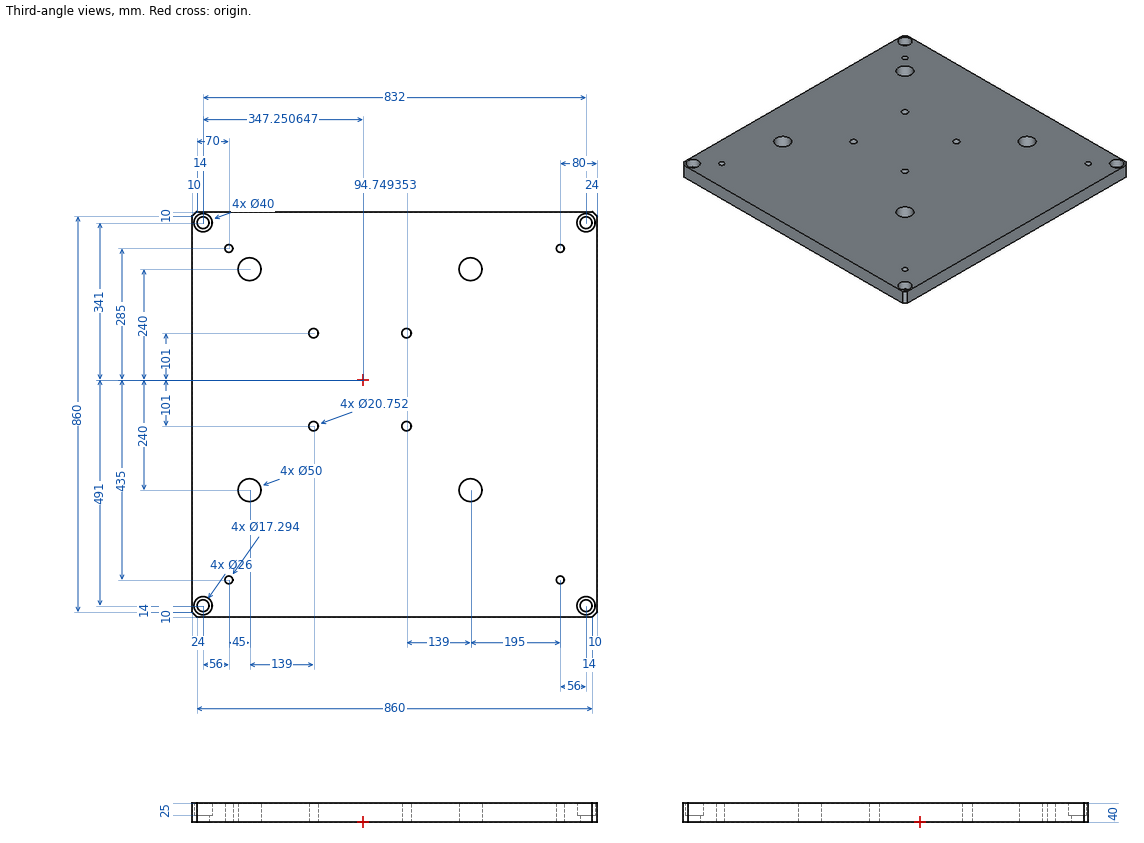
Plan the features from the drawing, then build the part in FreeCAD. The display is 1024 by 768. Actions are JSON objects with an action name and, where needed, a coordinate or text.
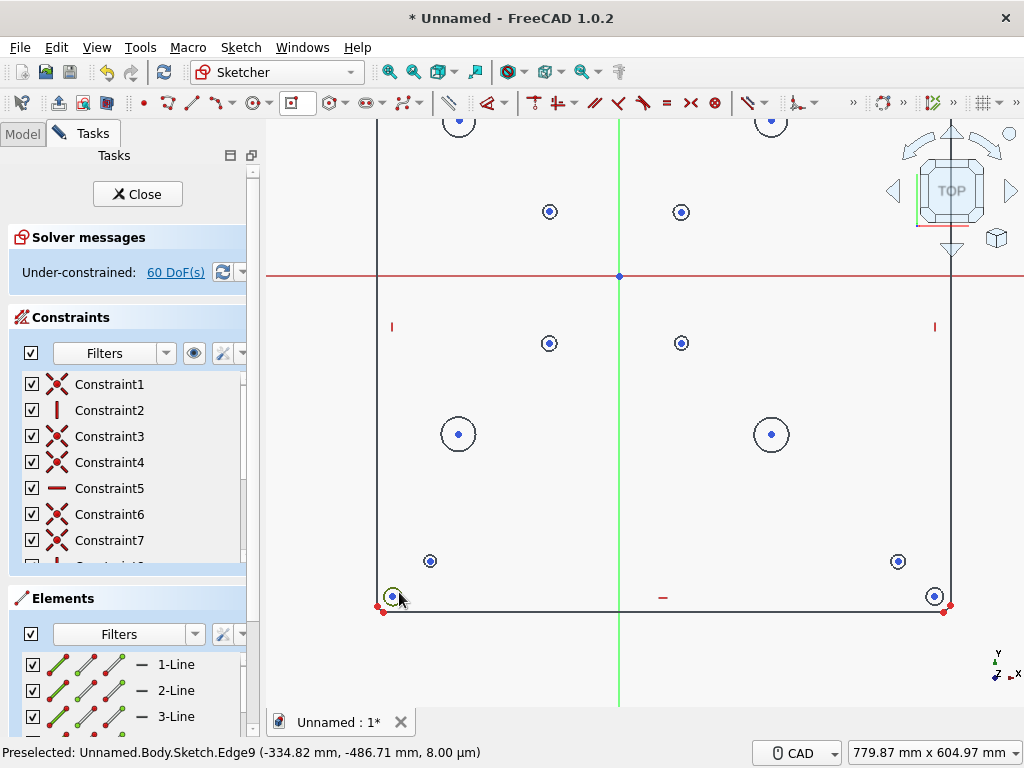
{"action": "scroll", "coordinate": [762, 591], "scroll_direction": "up", "scroll_amount": 5}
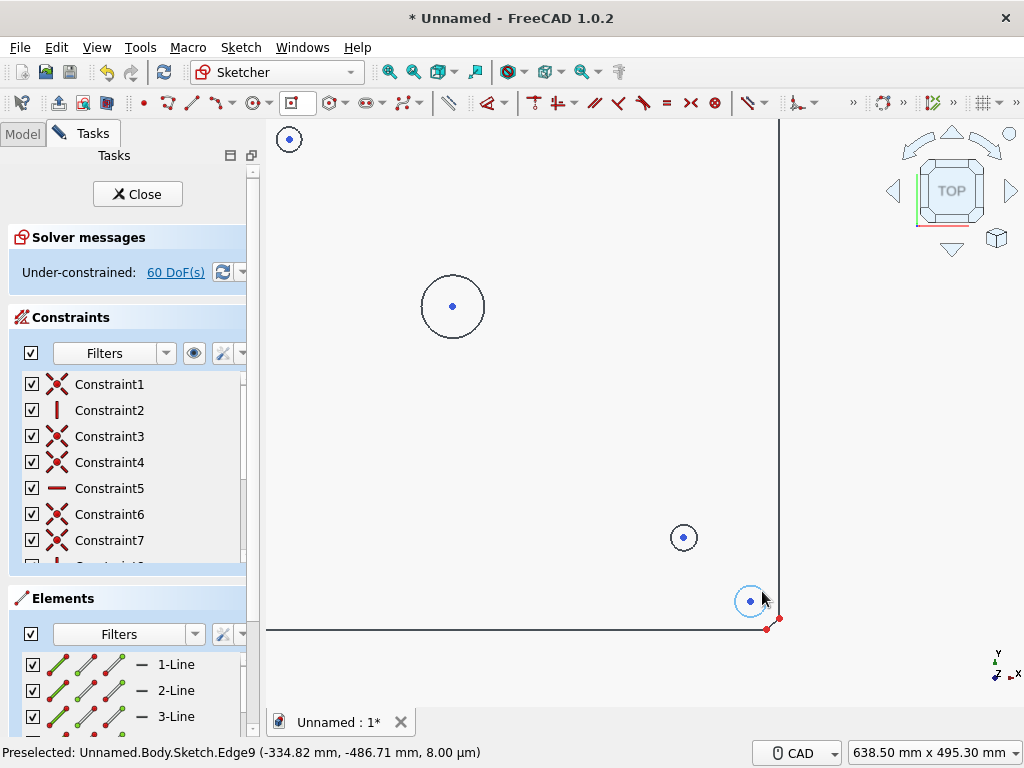
{"action": "left_click", "coordinate": [762, 590]}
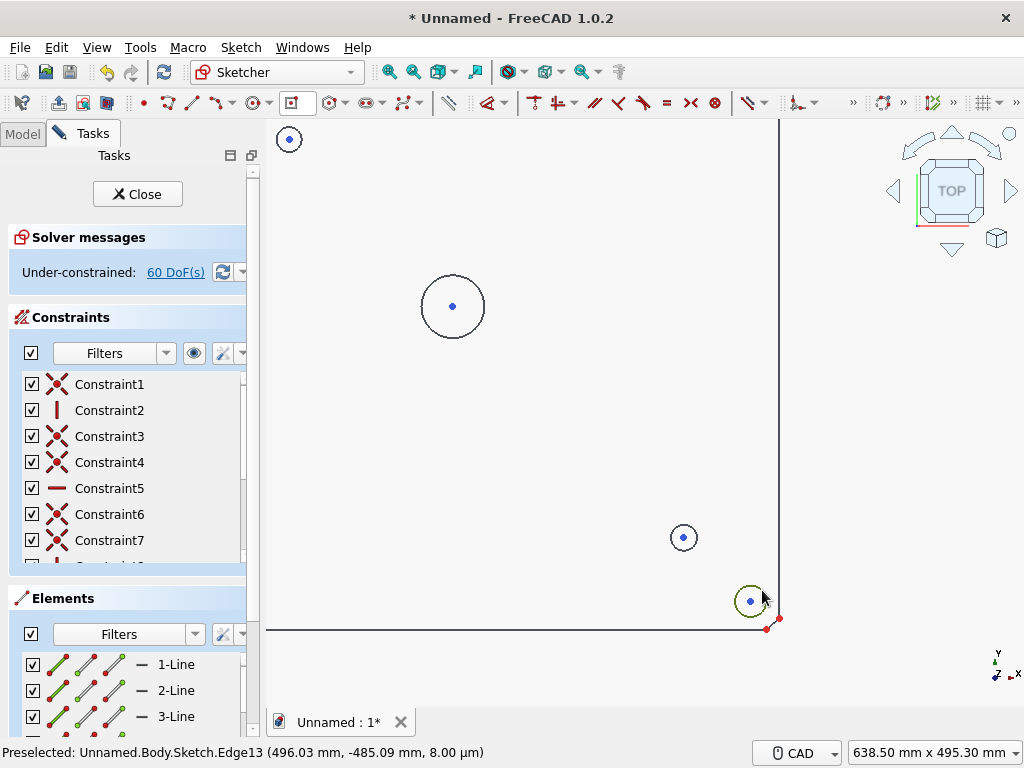
{"action": "scroll", "coordinate": [762, 591], "scroll_direction": "down", "scroll_amount": 5}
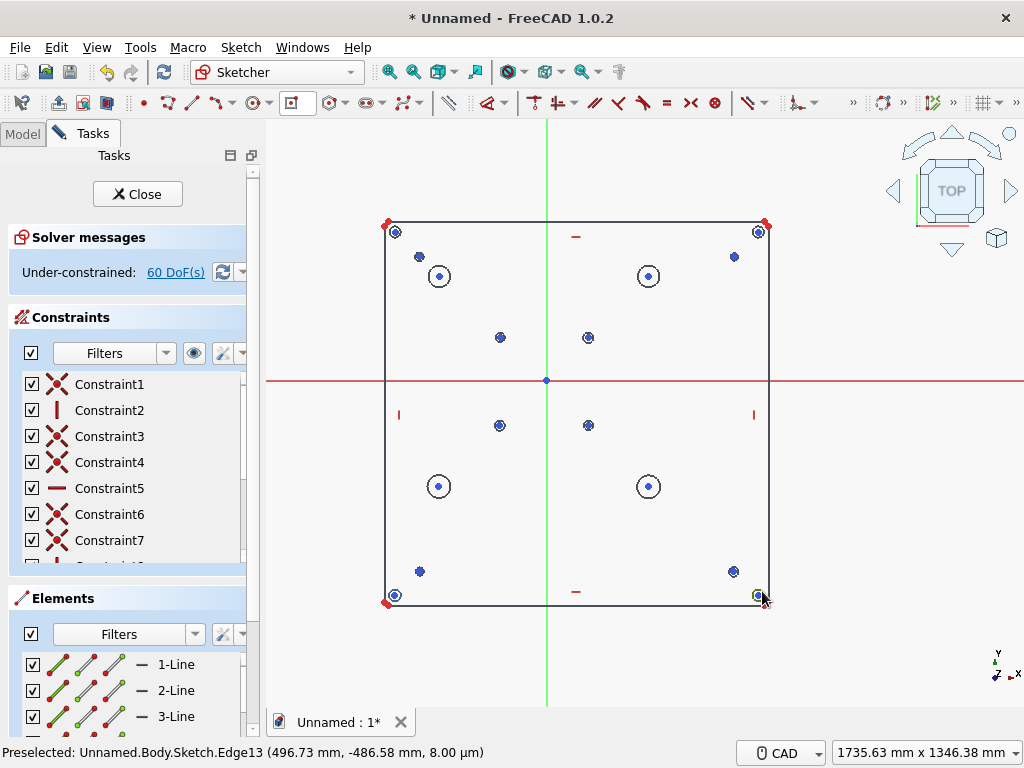
{"action": "scroll", "coordinate": [399, 228], "scroll_direction": "up", "scroll_amount": 5}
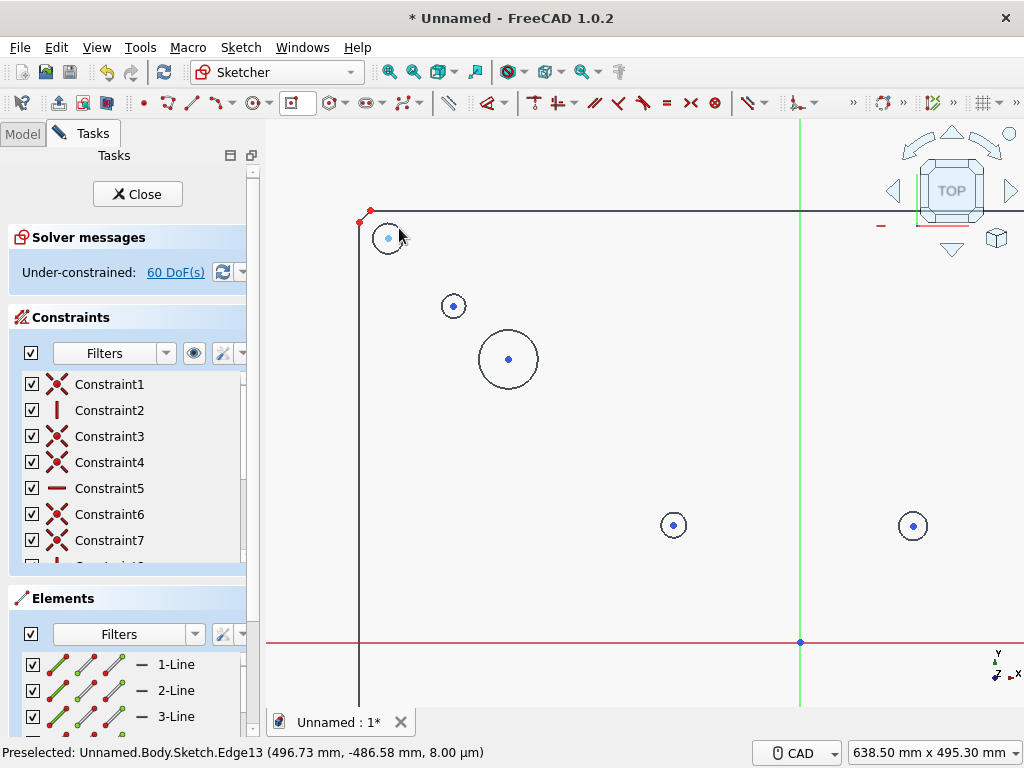
{"action": "left_click", "coordinate": [399, 228]}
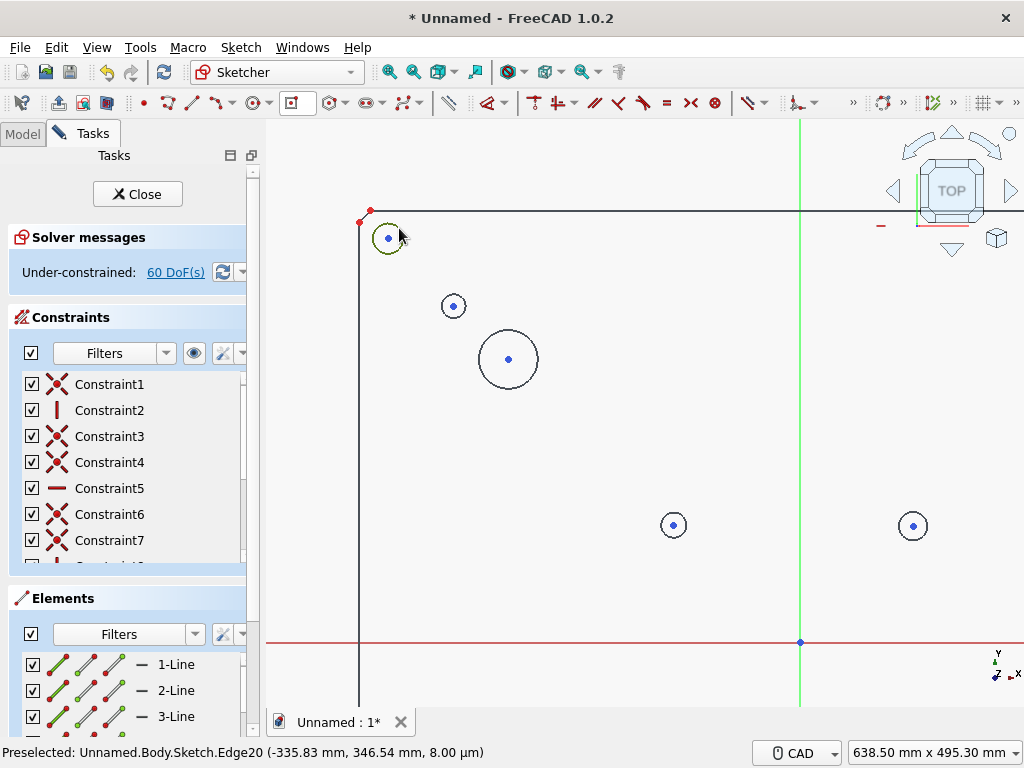
{"action": "scroll", "coordinate": [399, 227], "scroll_direction": "down", "scroll_amount": 5}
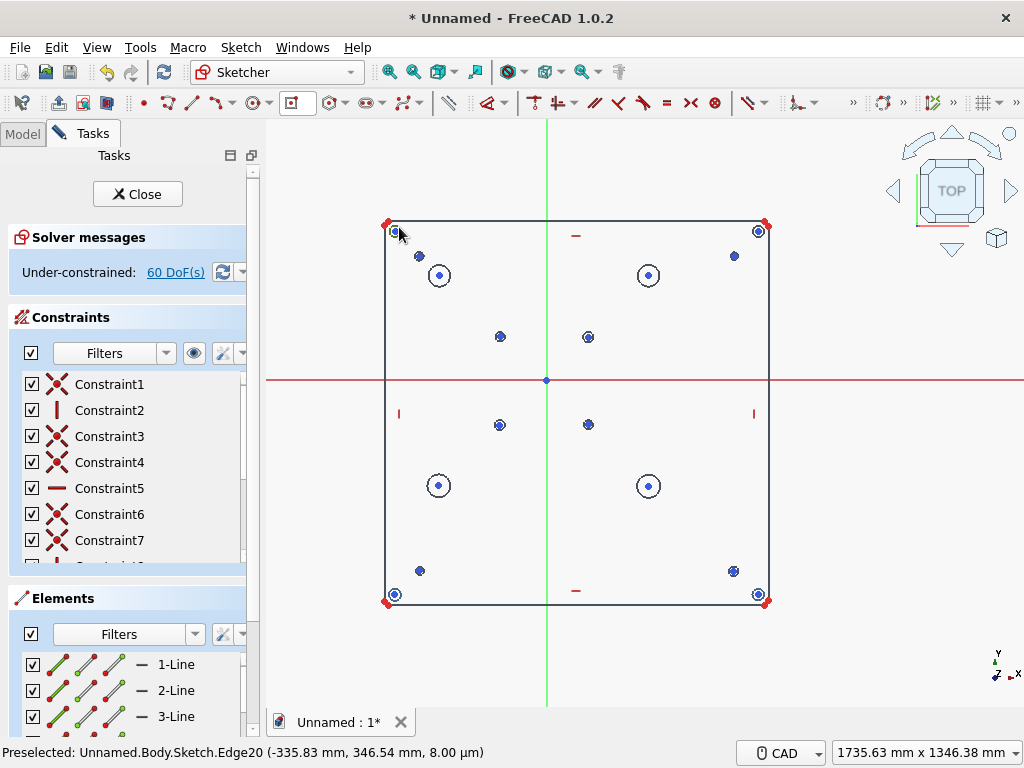
{"action": "scroll", "coordinate": [762, 227], "scroll_direction": "up", "scroll_amount": 5}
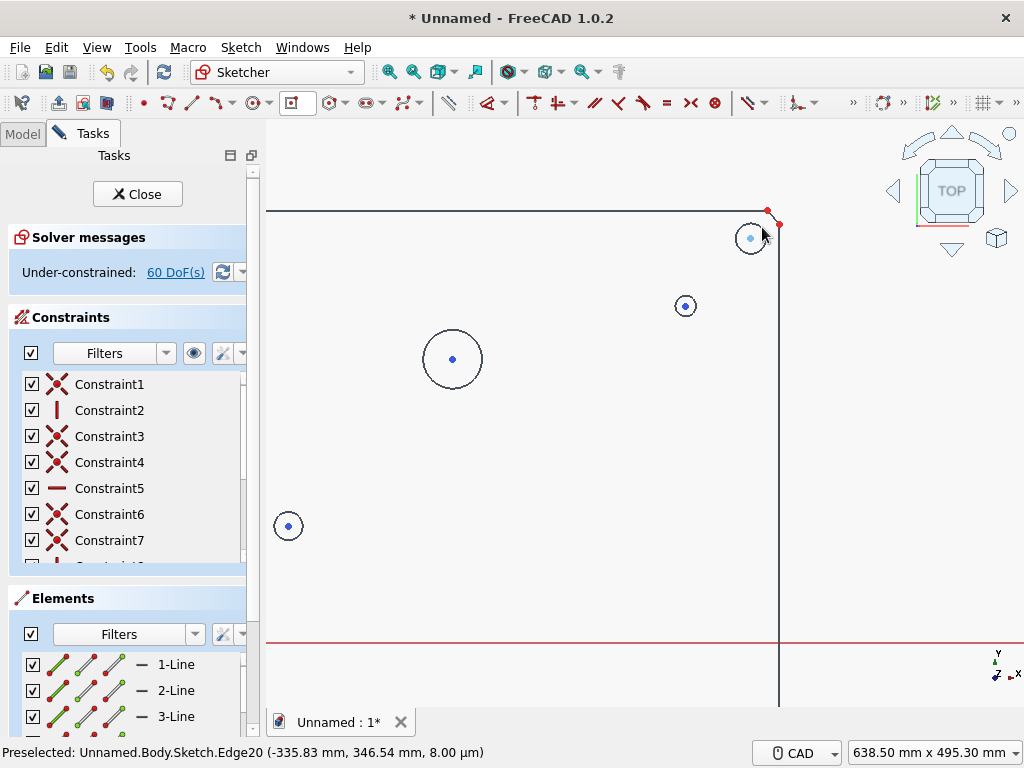
{"action": "left_click", "coordinate": [762, 228]}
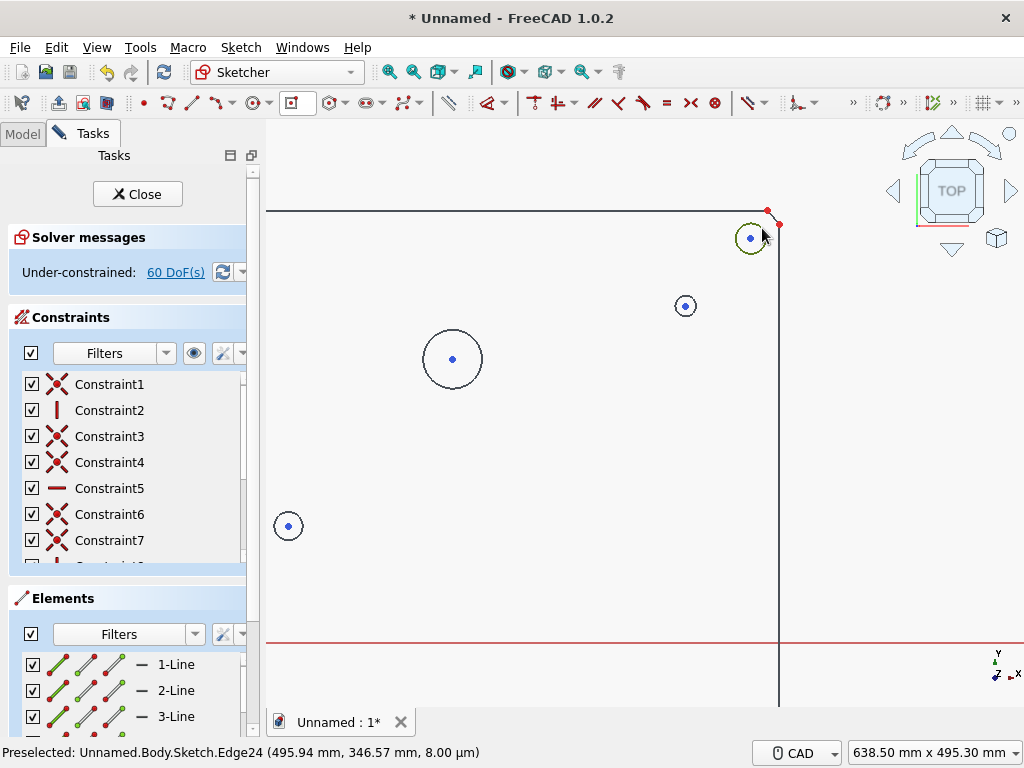
{"action": "key", "text": "e"}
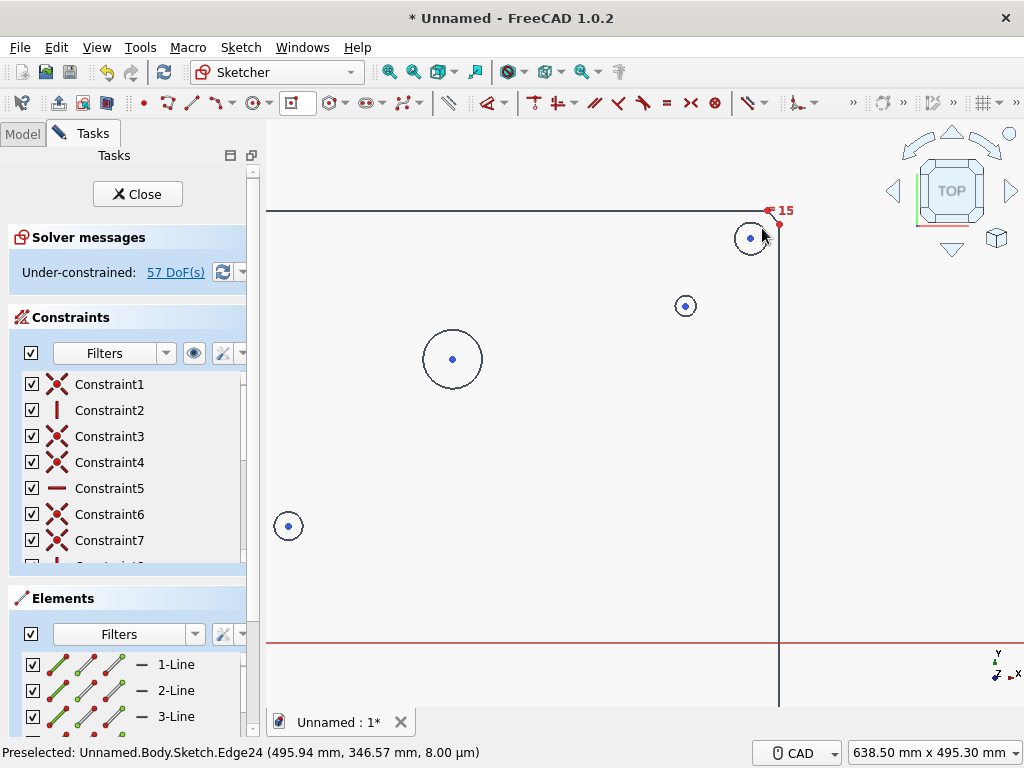
{"action": "scroll", "coordinate": [762, 227], "scroll_direction": "down", "scroll_amount": 5}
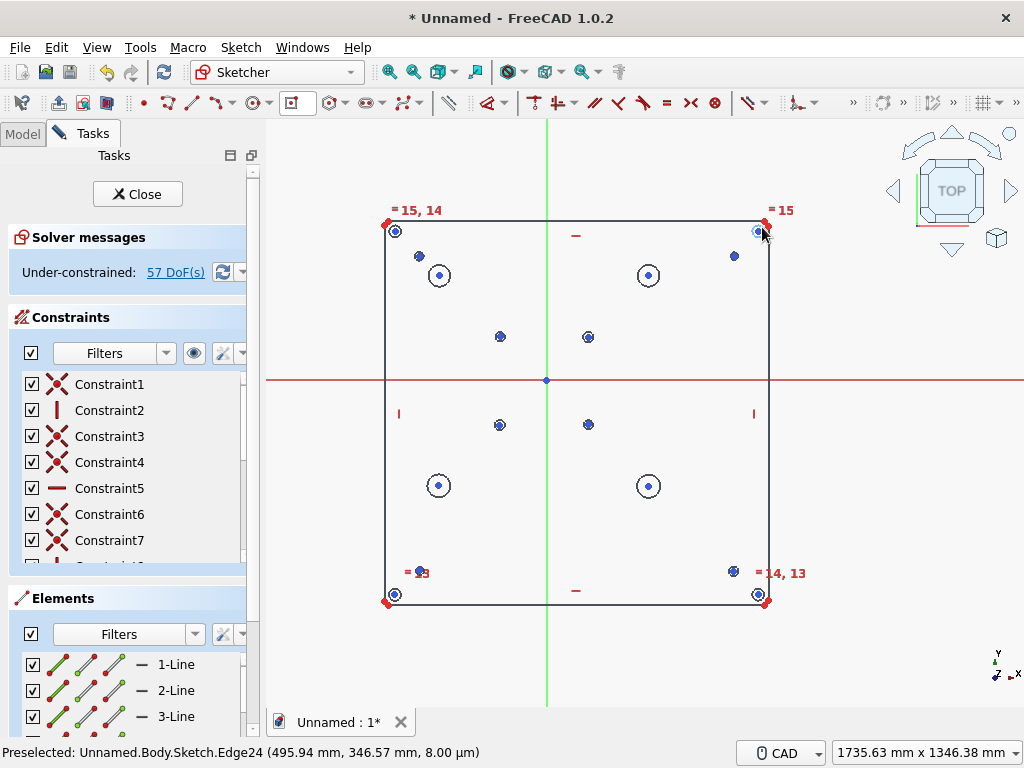
{"action": "scroll", "coordinate": [423, 568], "scroll_direction": "up", "scroll_amount": 7}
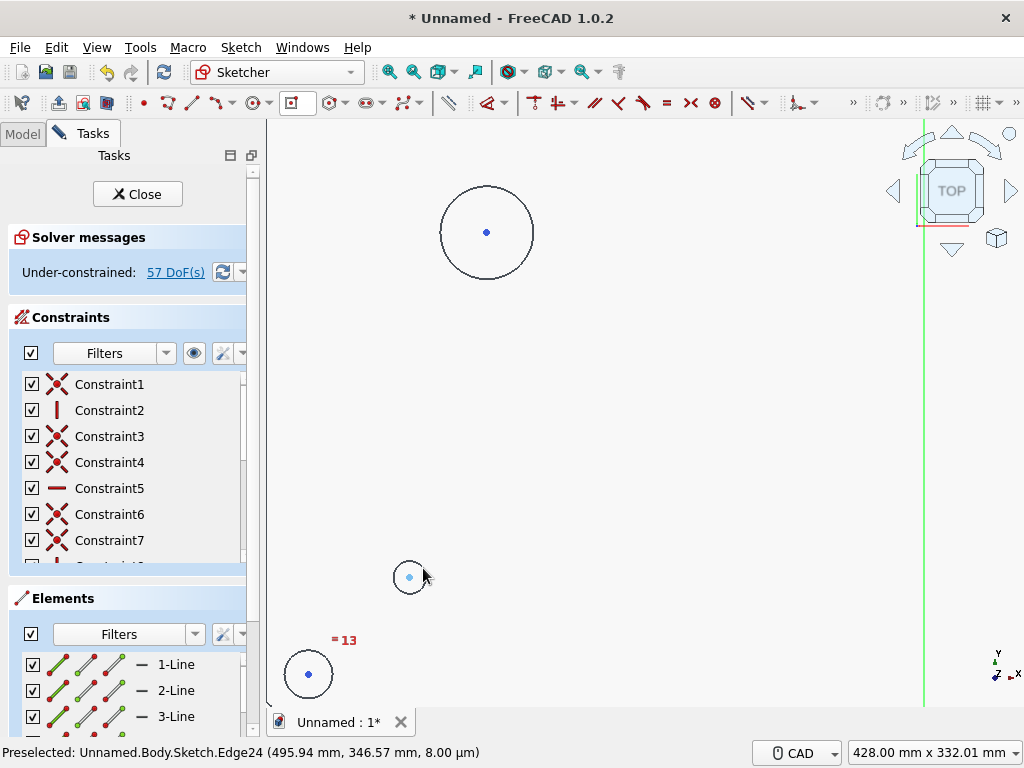
{"action": "left_click", "coordinate": [421, 566]}